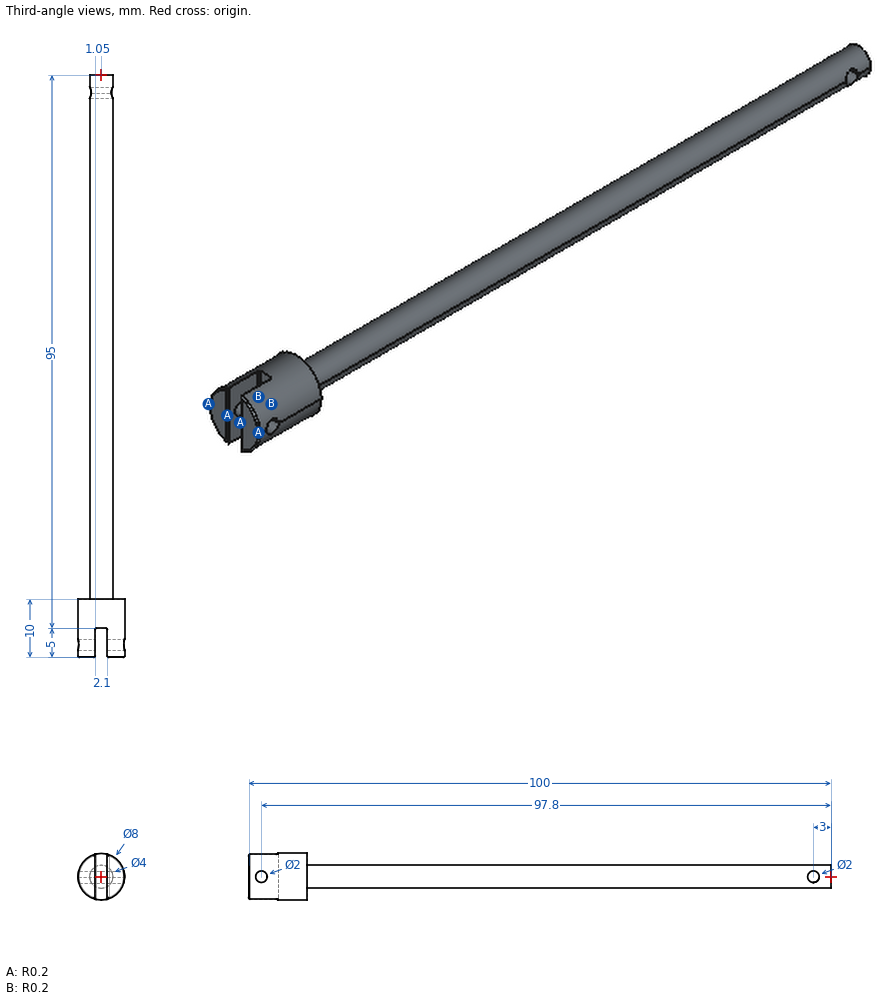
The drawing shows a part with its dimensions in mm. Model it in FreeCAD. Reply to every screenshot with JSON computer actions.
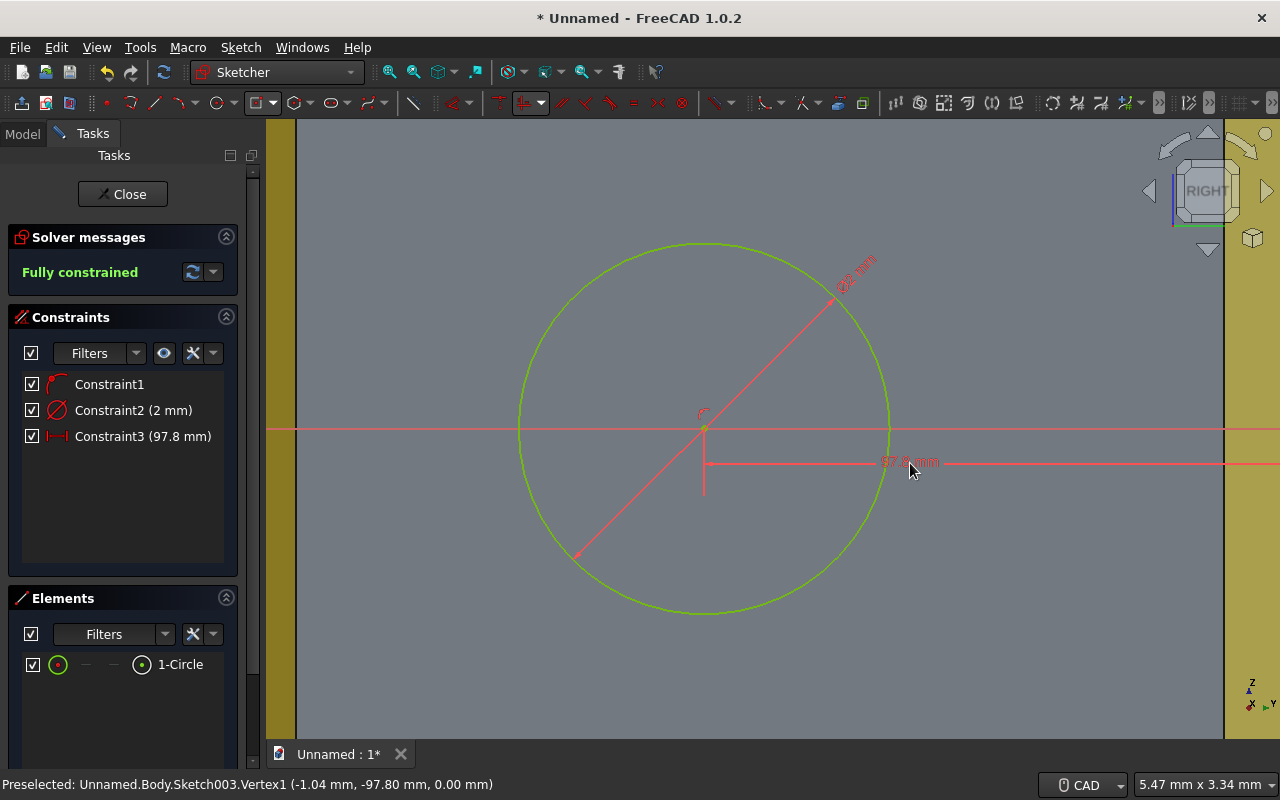
{"action": "left_click", "coordinate": [123, 194]}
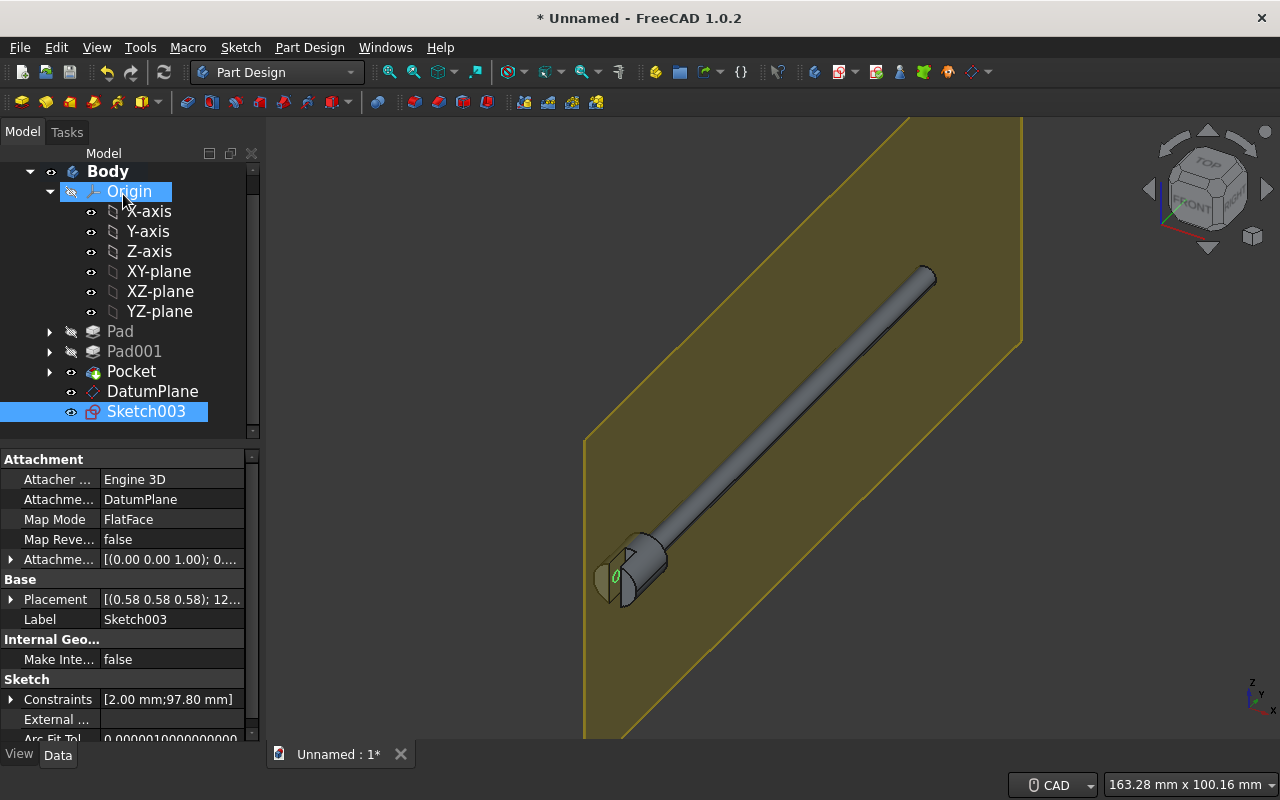
{"action": "left_click", "coordinate": [188, 102]}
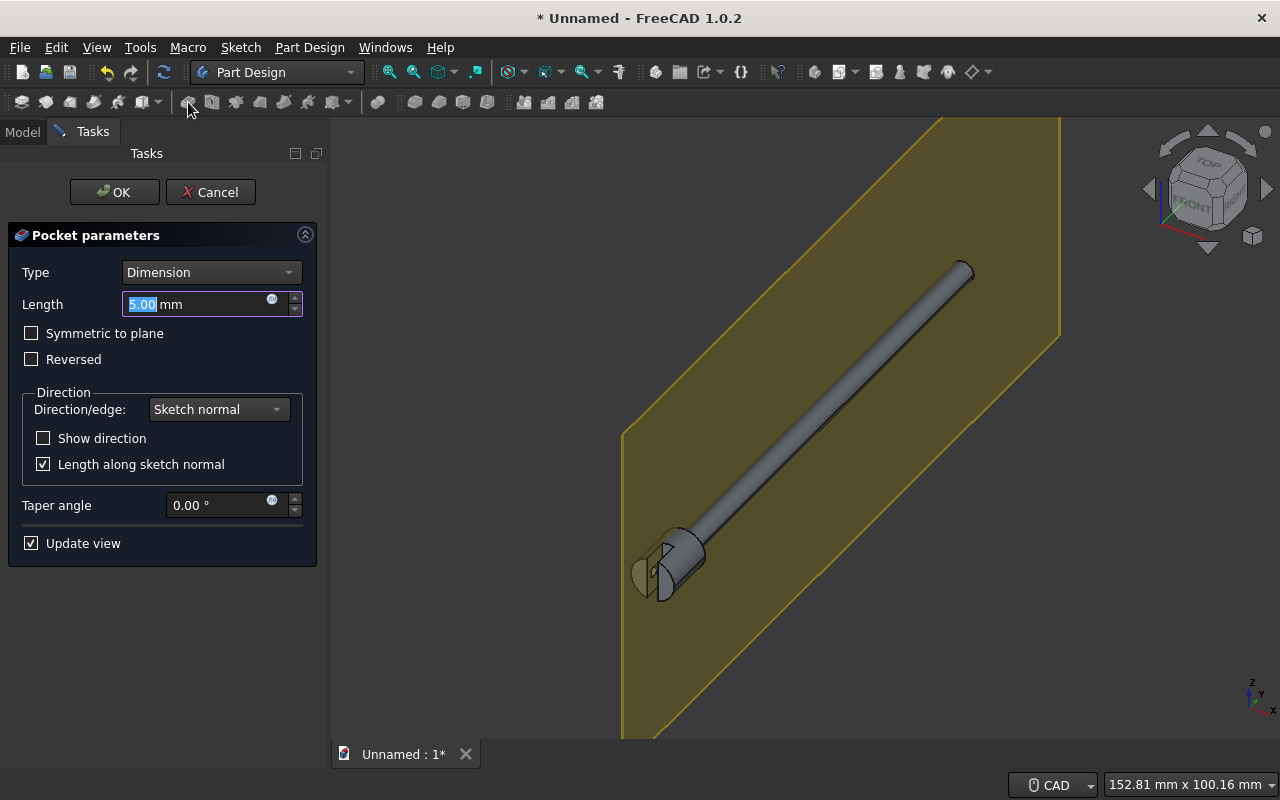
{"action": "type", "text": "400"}
{"action": "key", "text": "Tab"}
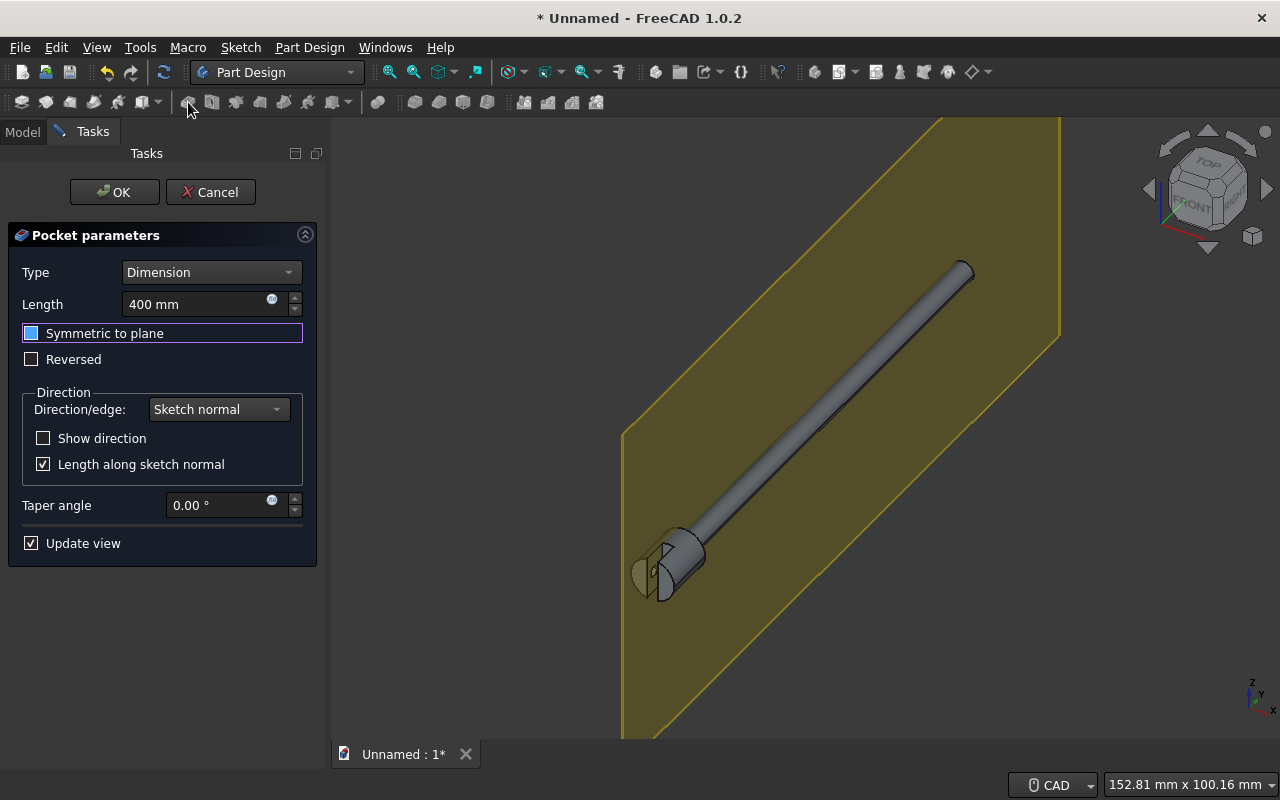
{"action": "left_click", "coordinate": [30, 333]}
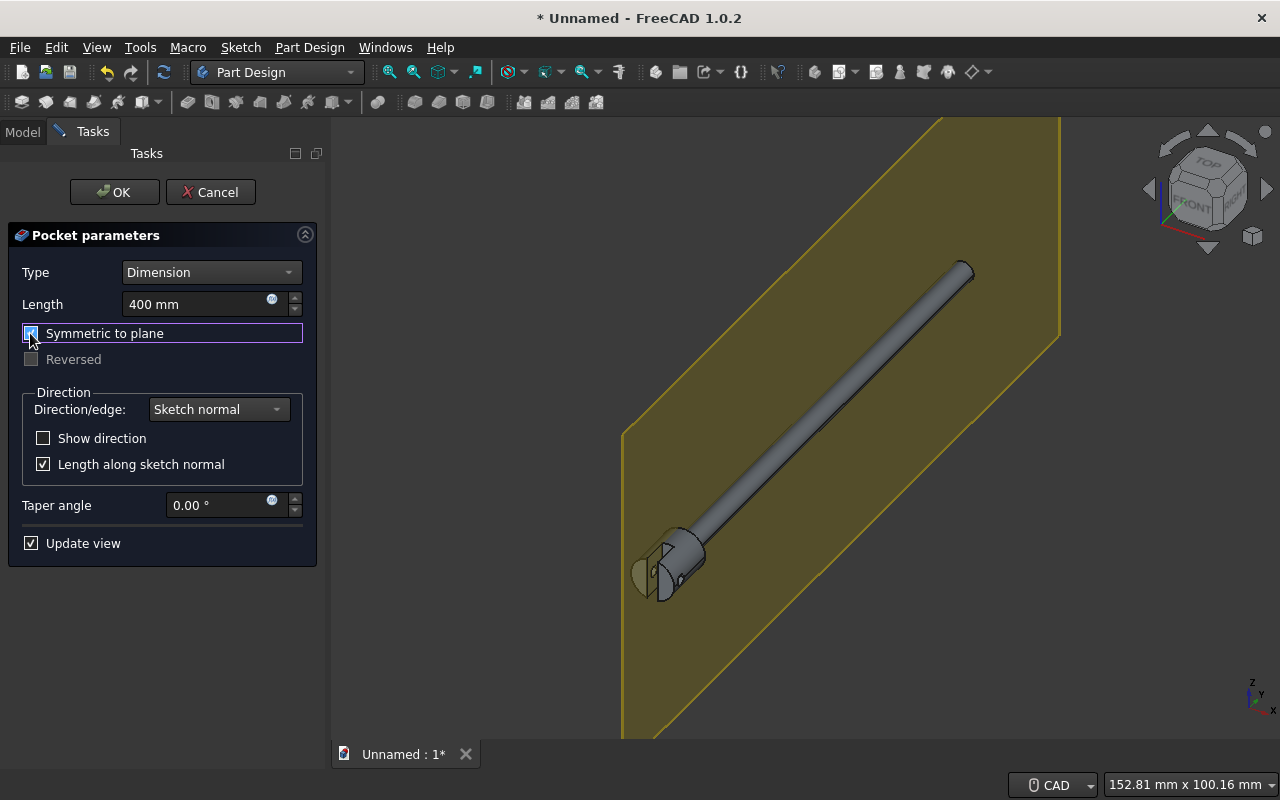
{"action": "left_click", "coordinate": [115, 192]}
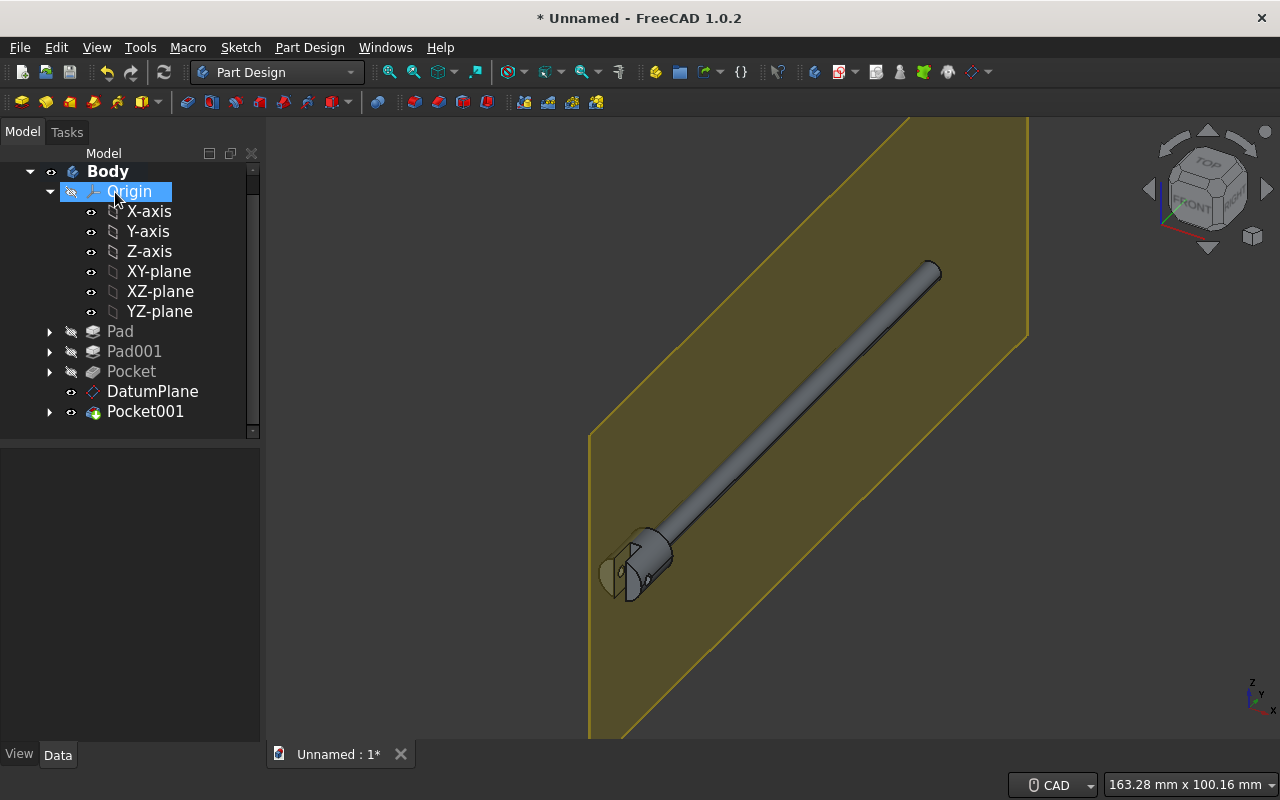
{"action": "left_click", "coordinate": [116, 392]}
{"action": "key", "text": "space"}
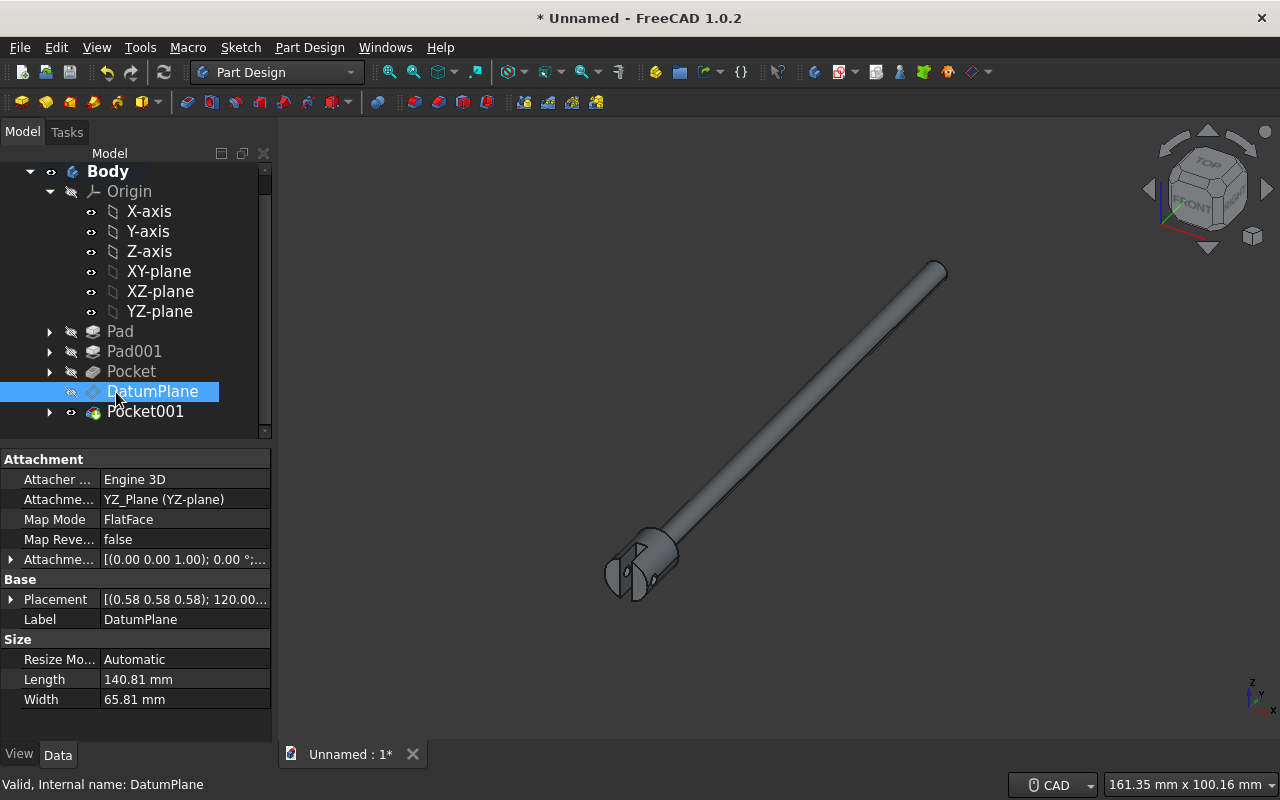
{"action": "left_click", "coordinate": [318, 699]}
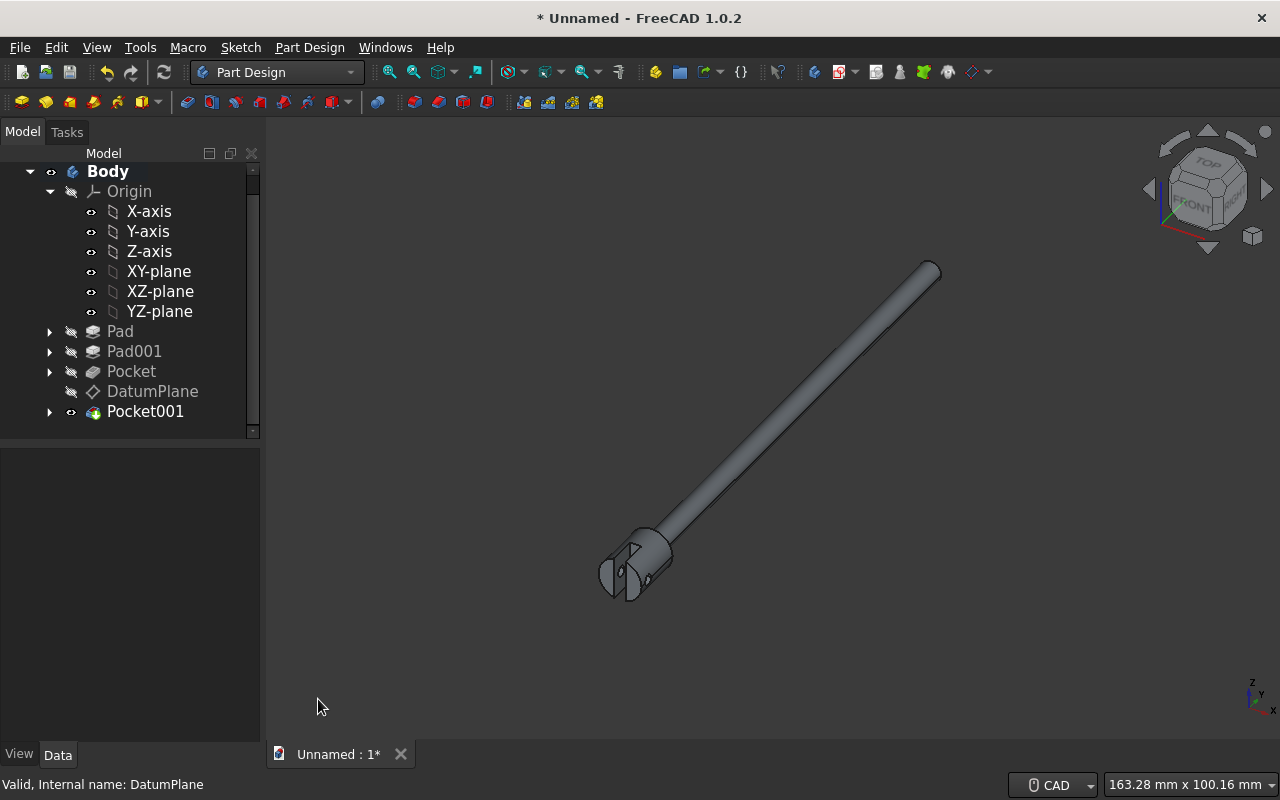
{"action": "left_click", "coordinate": [840, 72]}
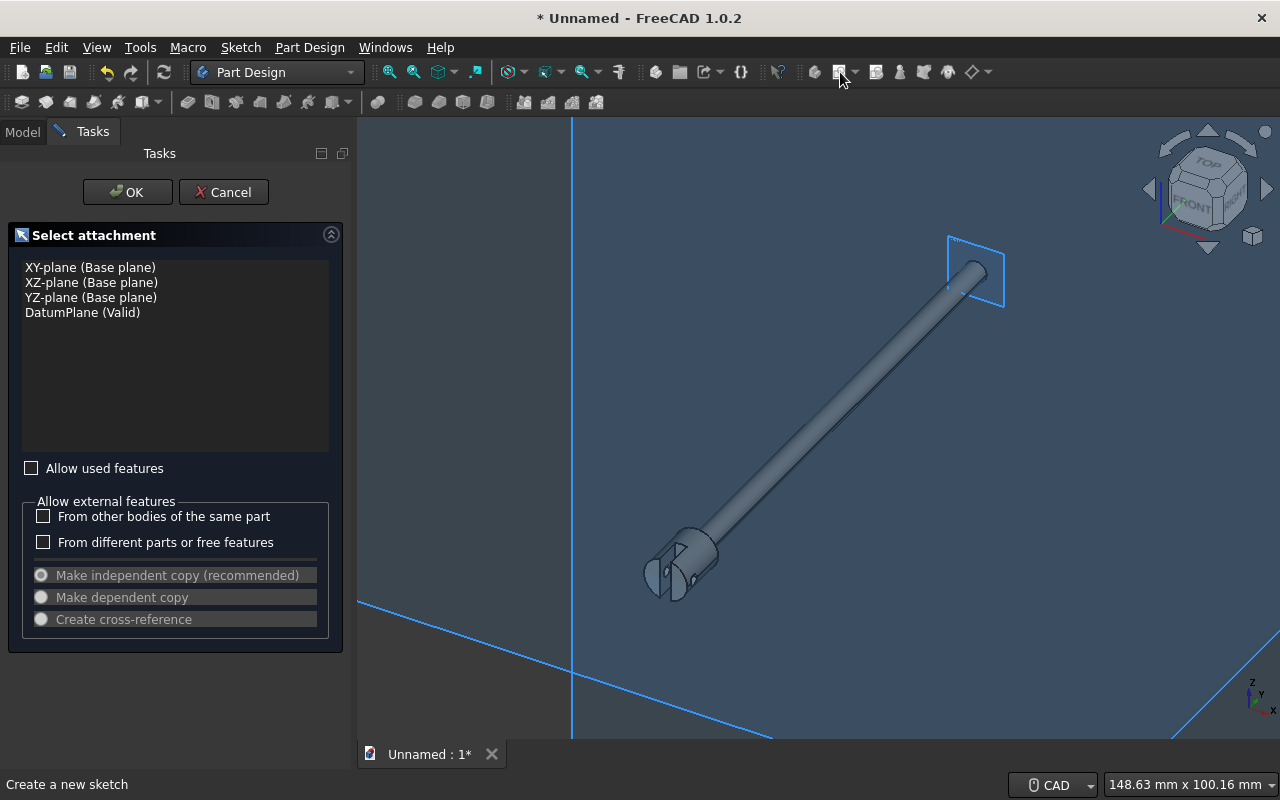
{"action": "left_click", "coordinate": [82, 298]}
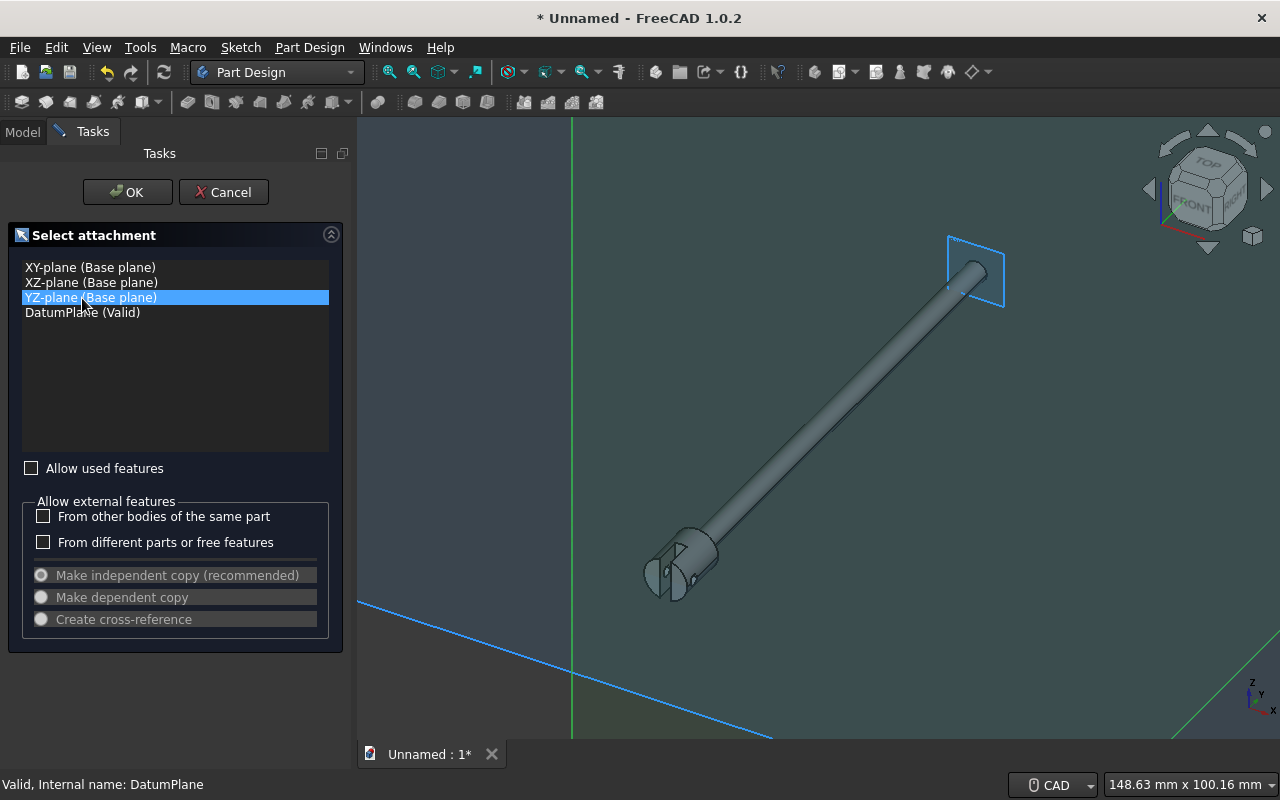
{"action": "left_click", "coordinate": [128, 192]}